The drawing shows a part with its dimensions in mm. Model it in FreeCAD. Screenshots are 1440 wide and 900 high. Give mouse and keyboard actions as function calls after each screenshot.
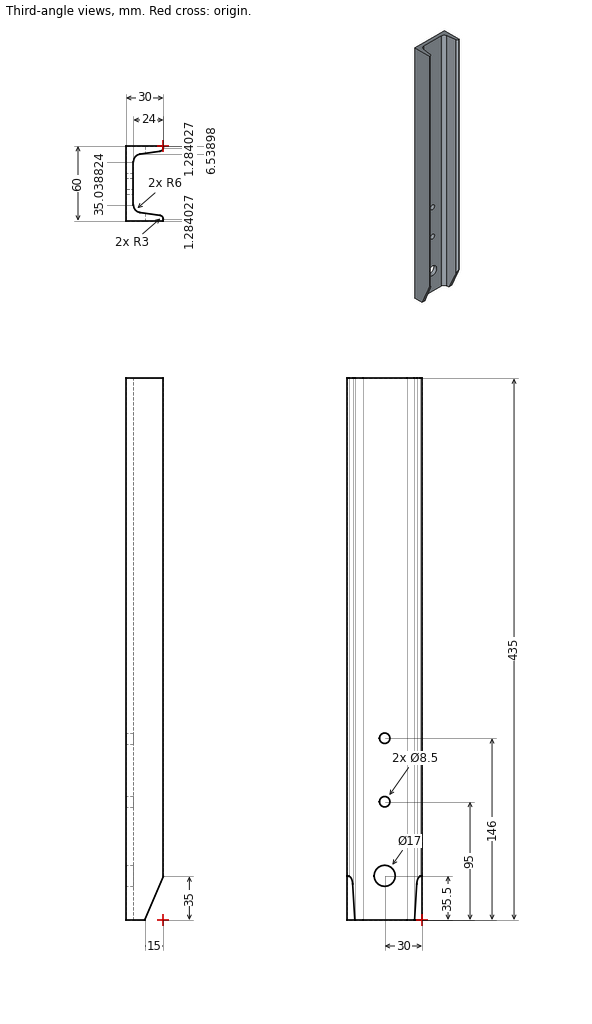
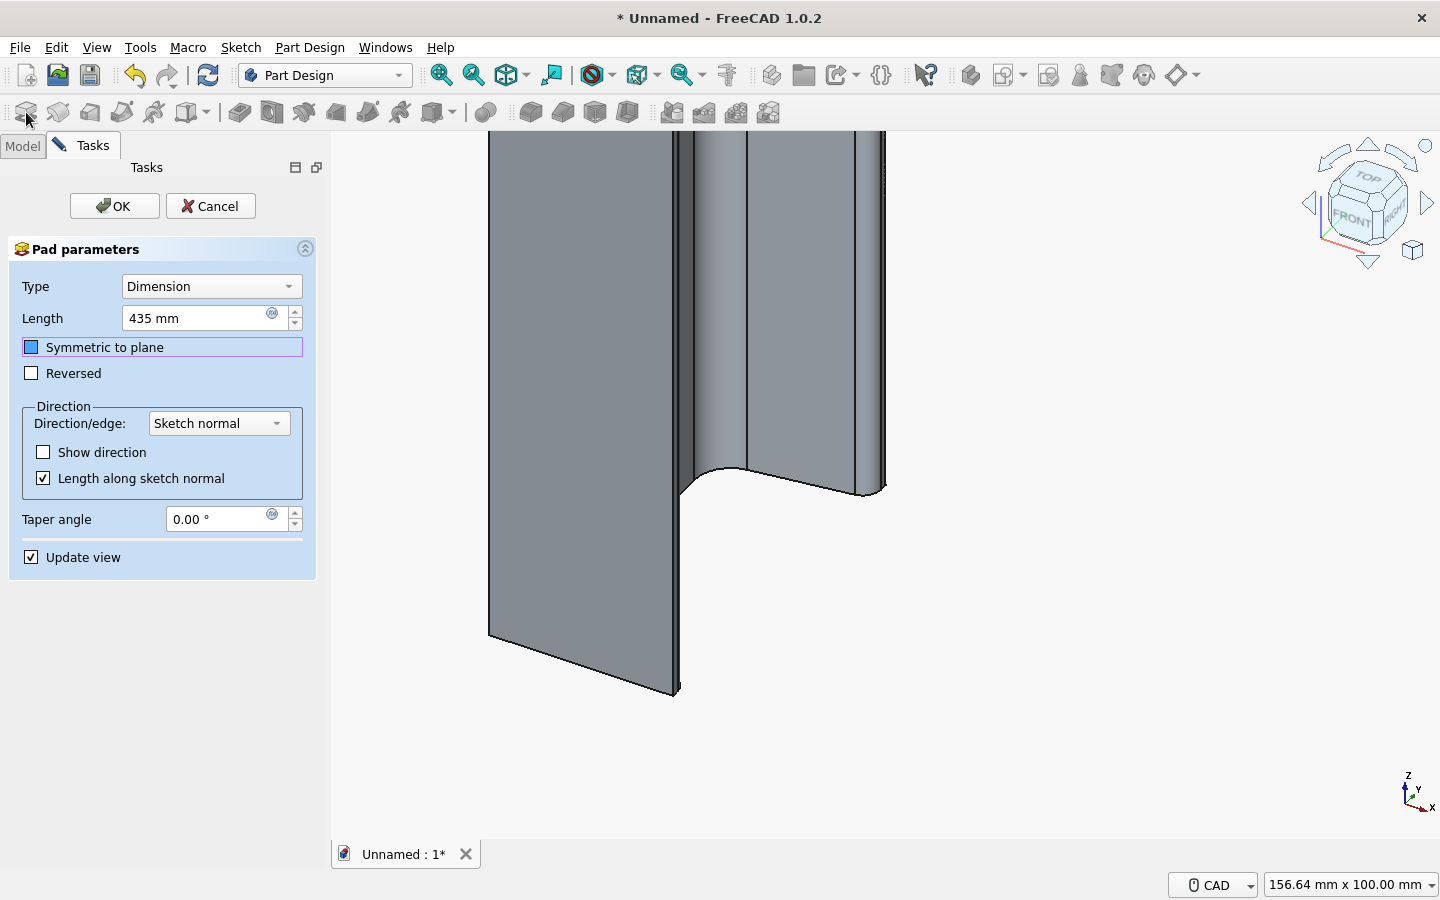
click(115, 206)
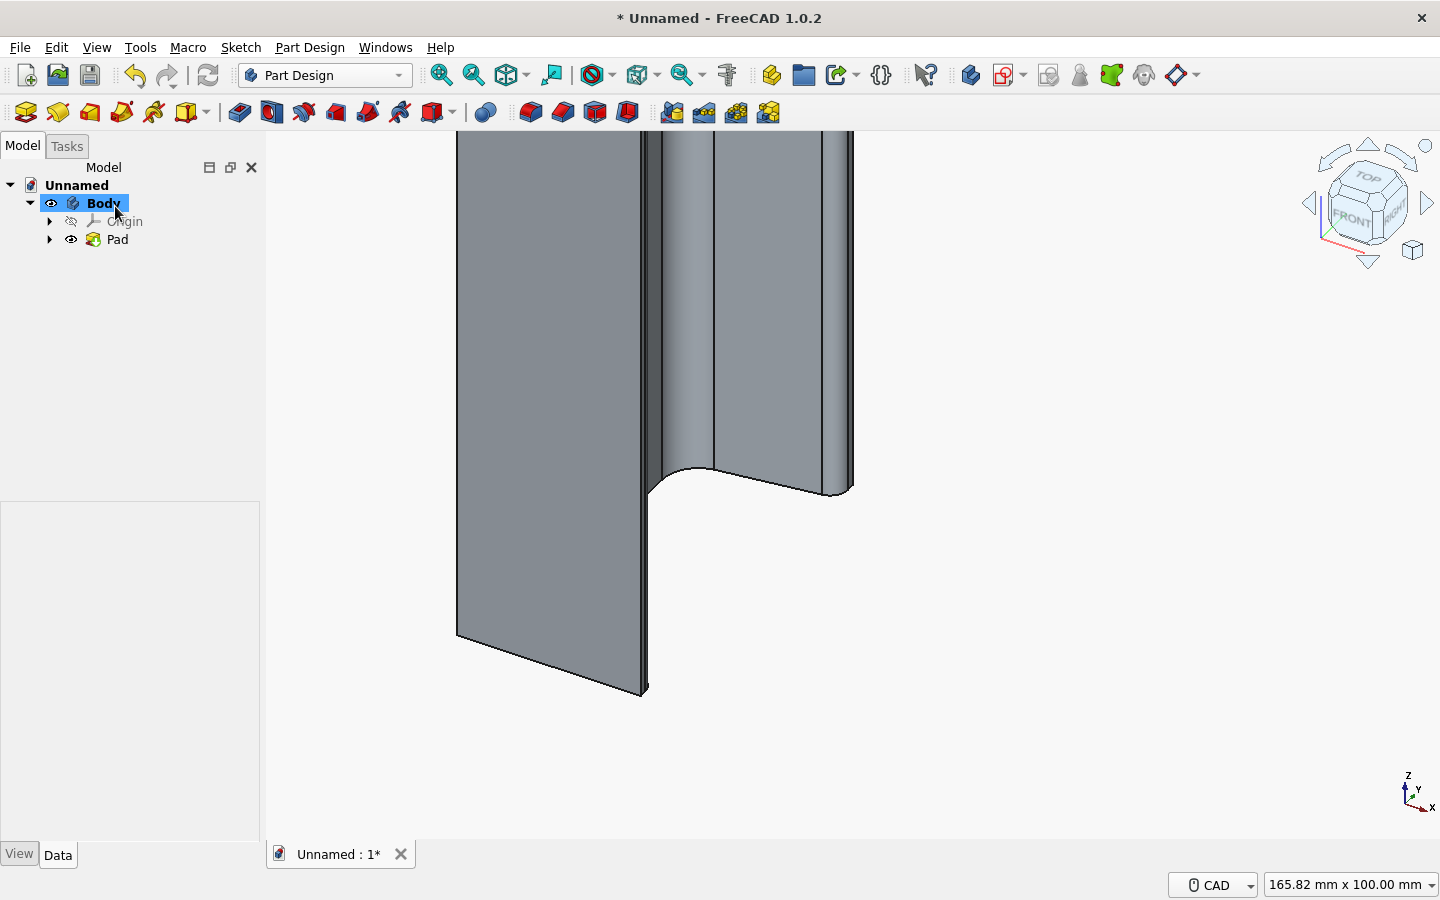
key(v)
key(f)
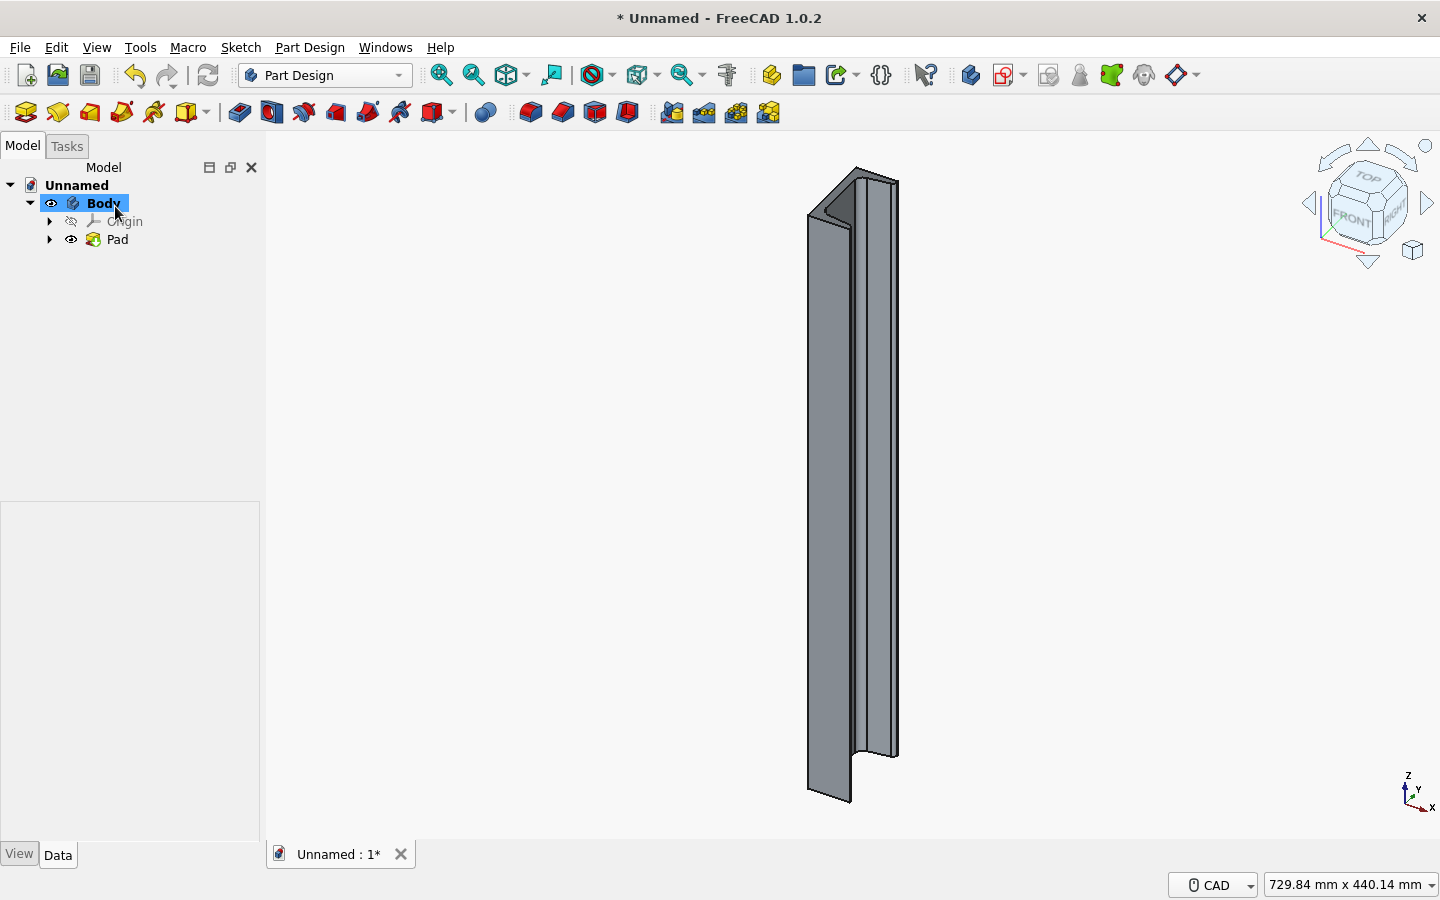
key(6)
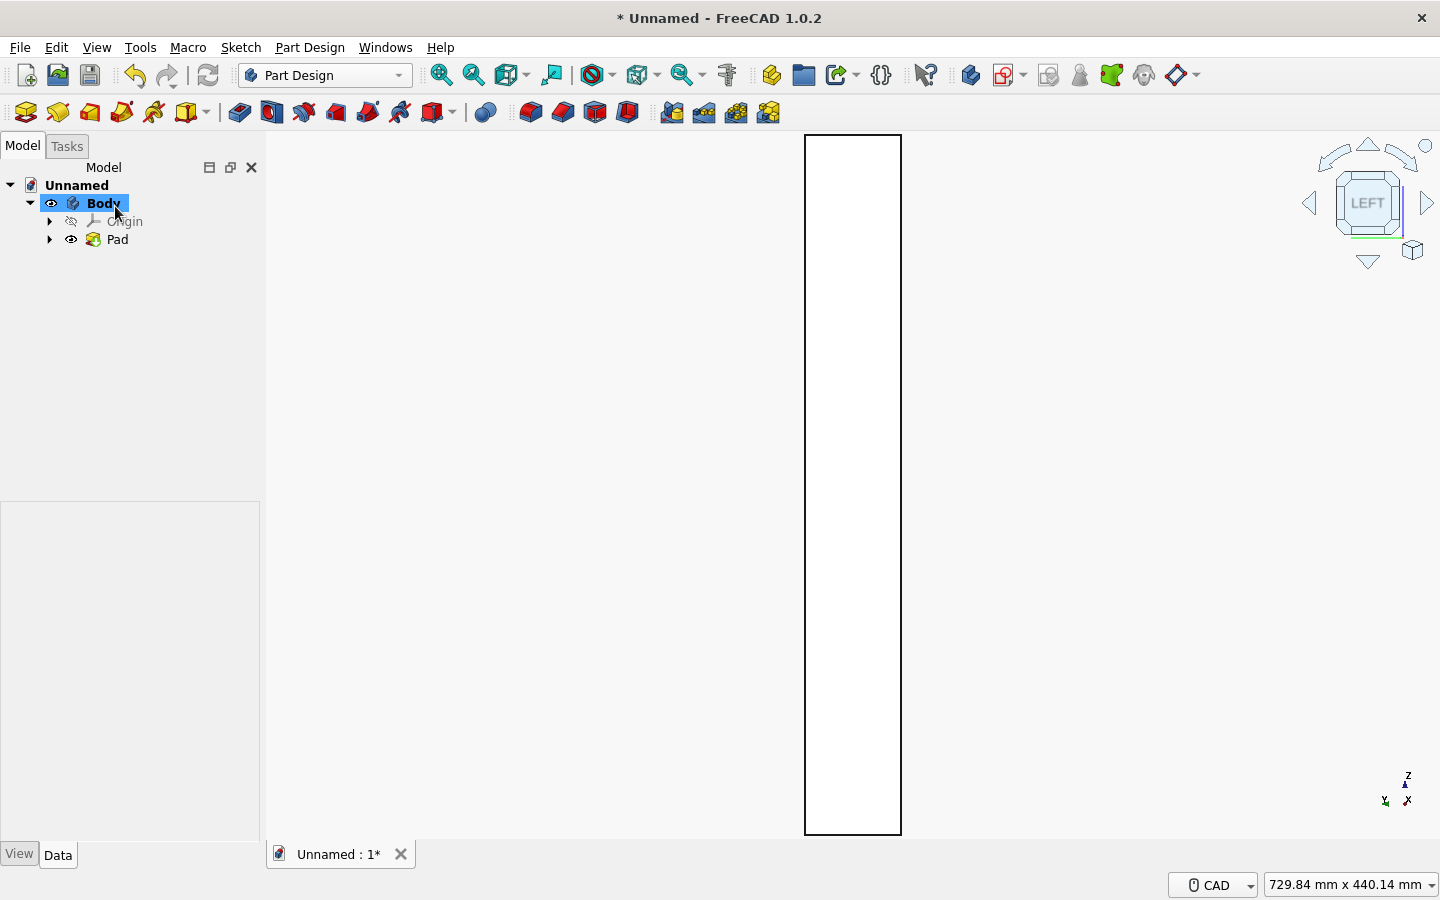
click(853, 184)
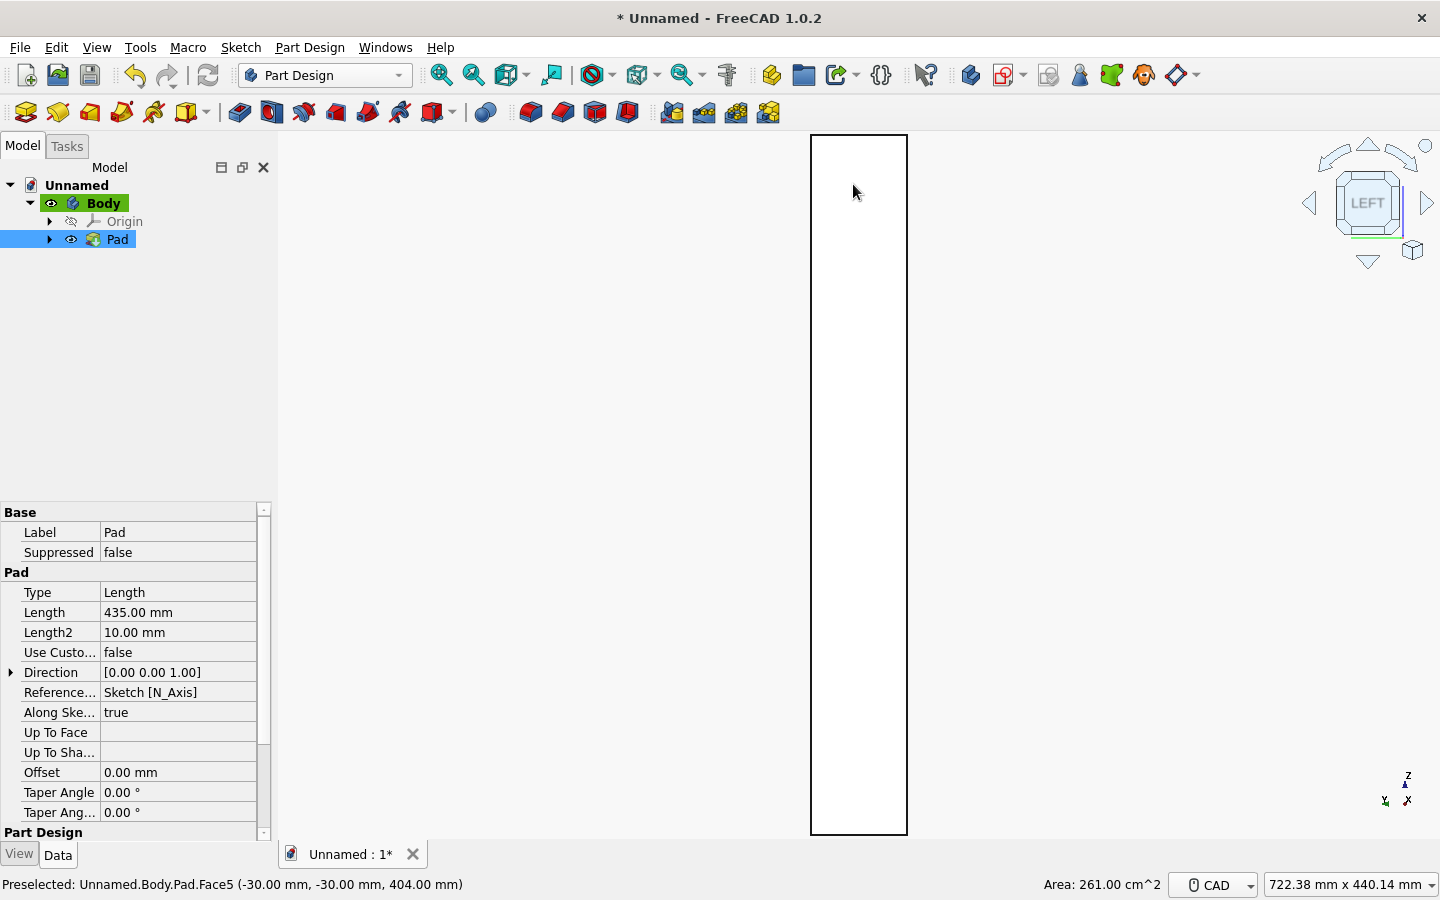
click(1004, 76)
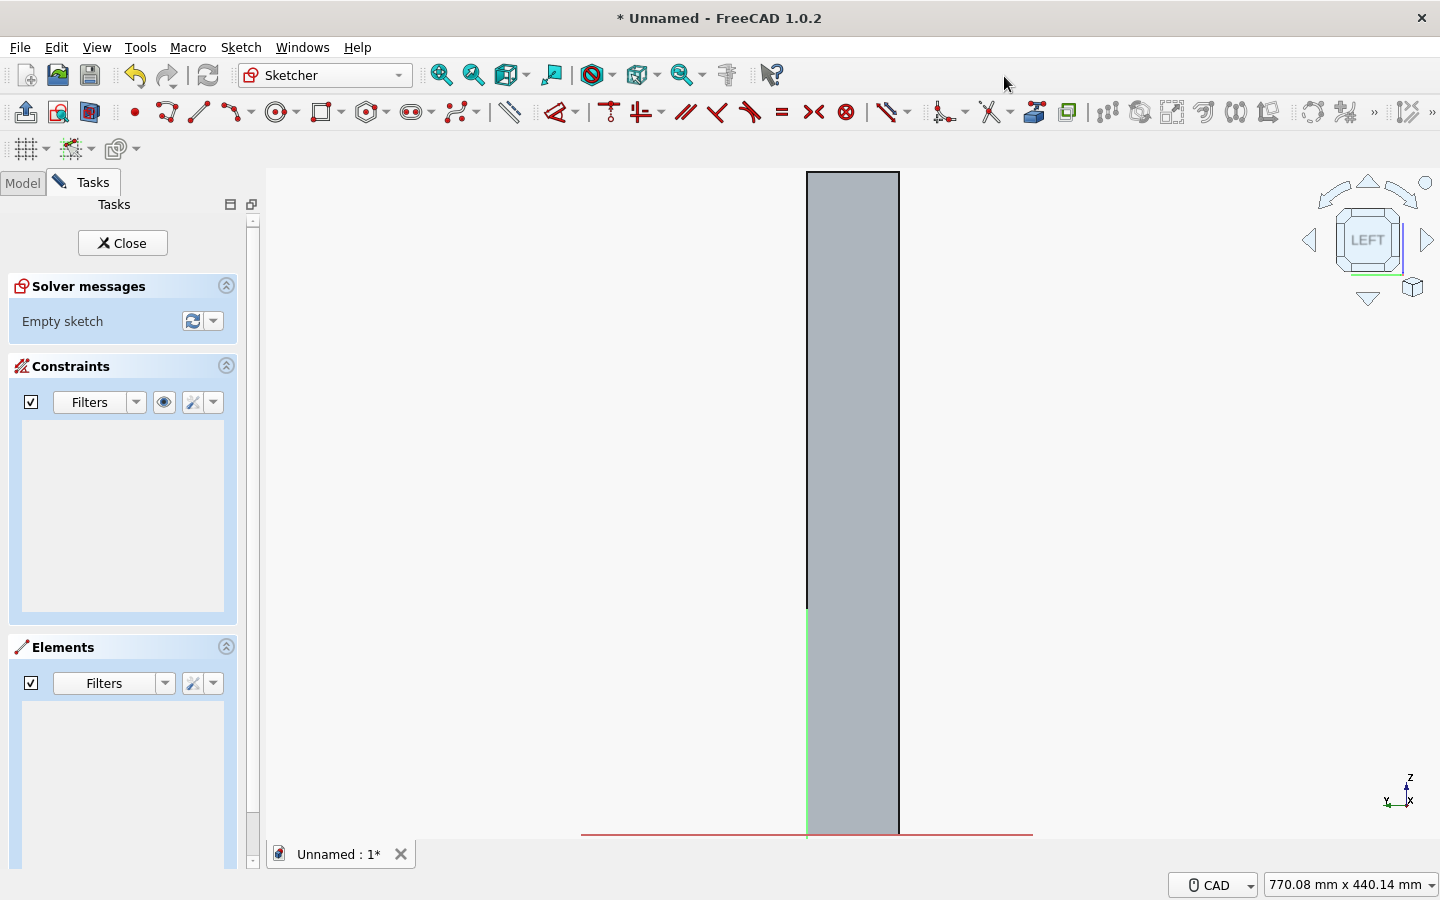
scroll(857, 799, up, 14)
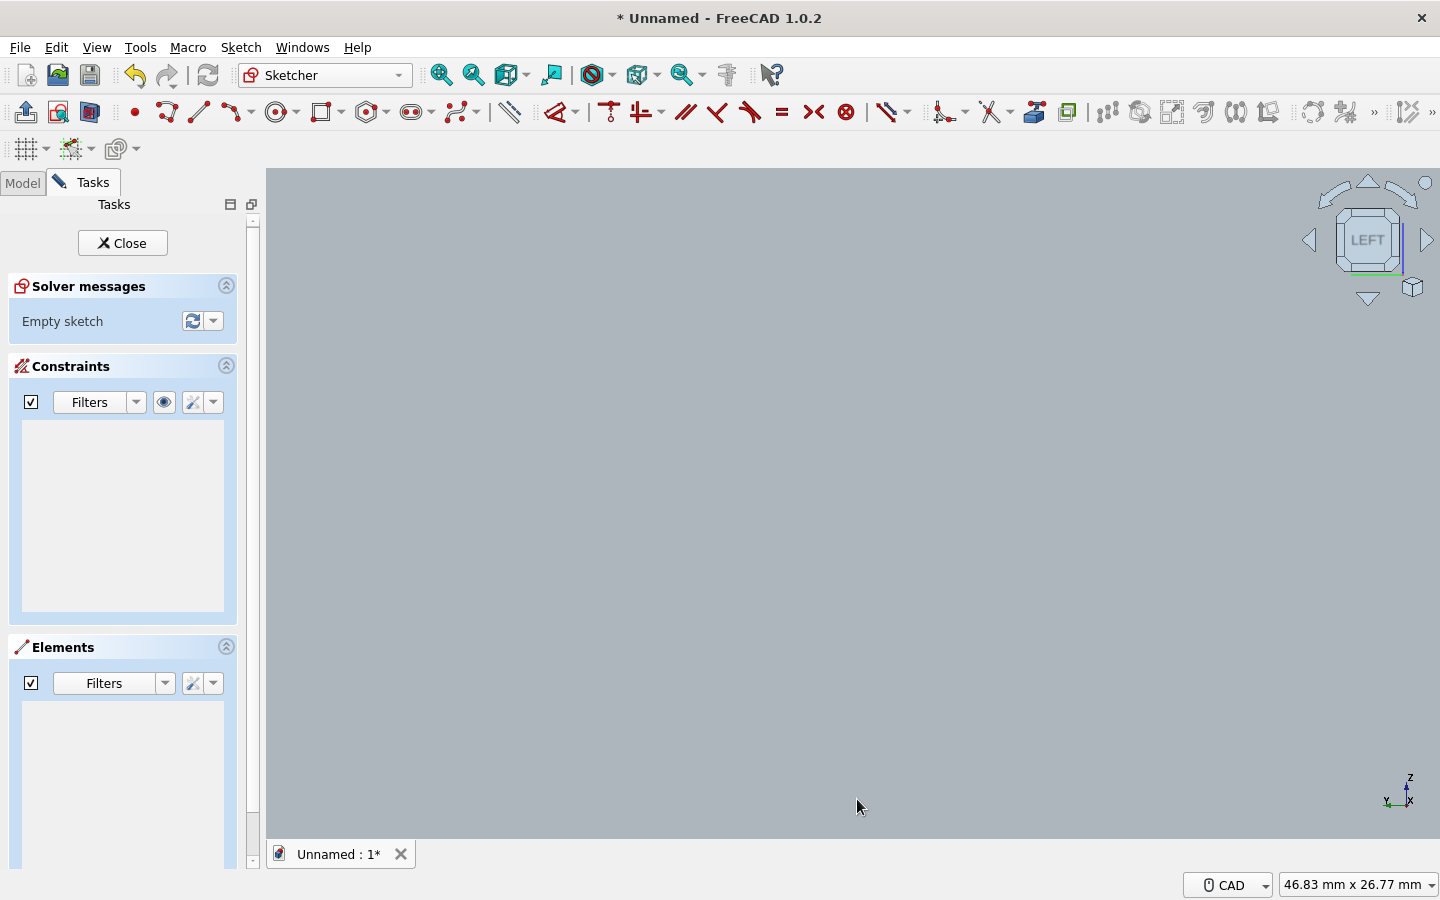
click(276, 112)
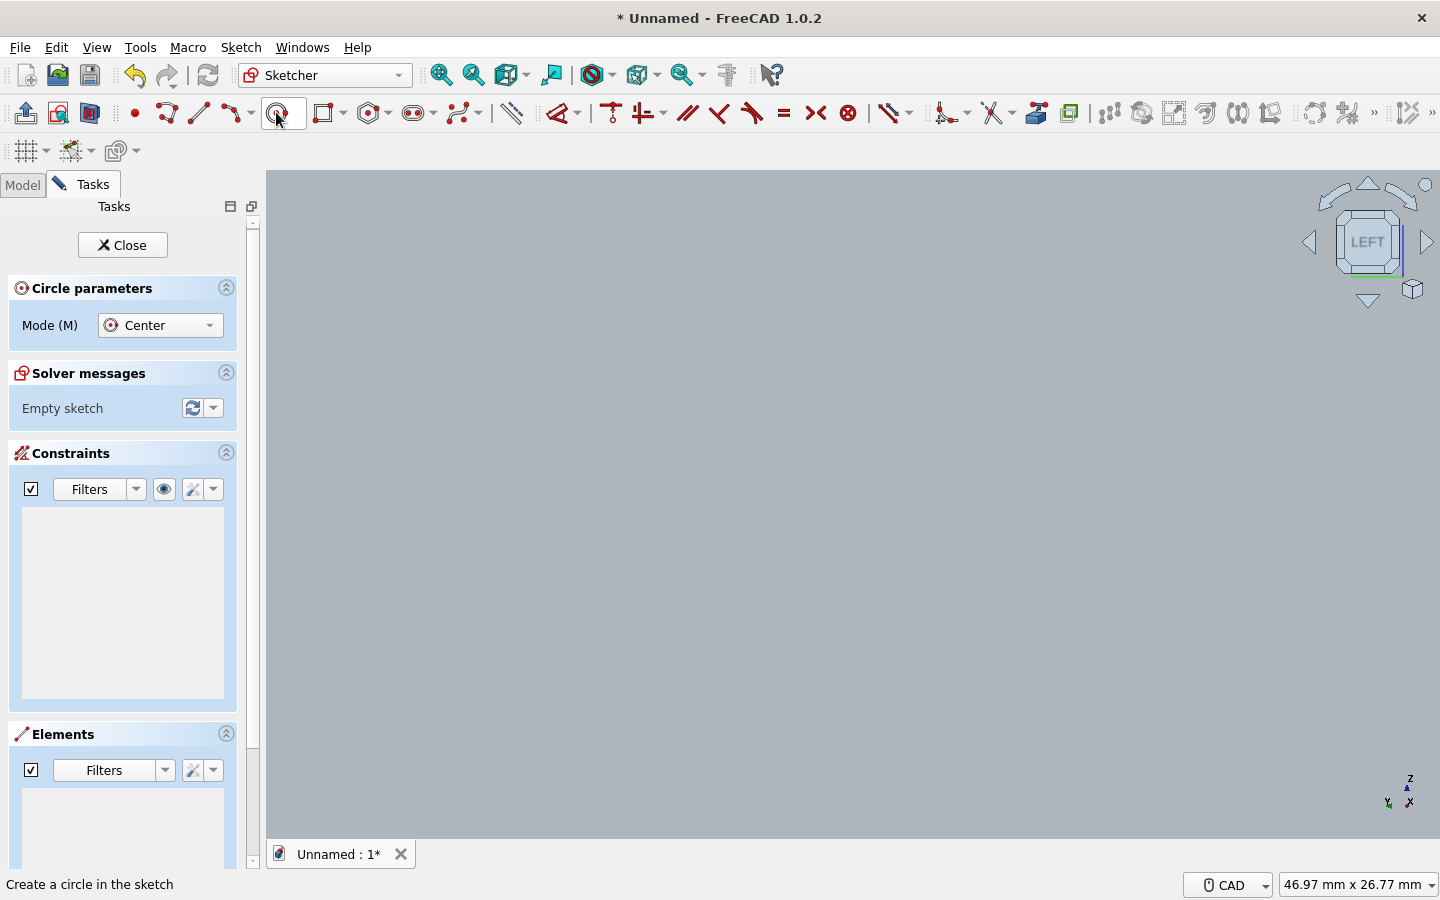
click(784, 489)
move(934, 339)